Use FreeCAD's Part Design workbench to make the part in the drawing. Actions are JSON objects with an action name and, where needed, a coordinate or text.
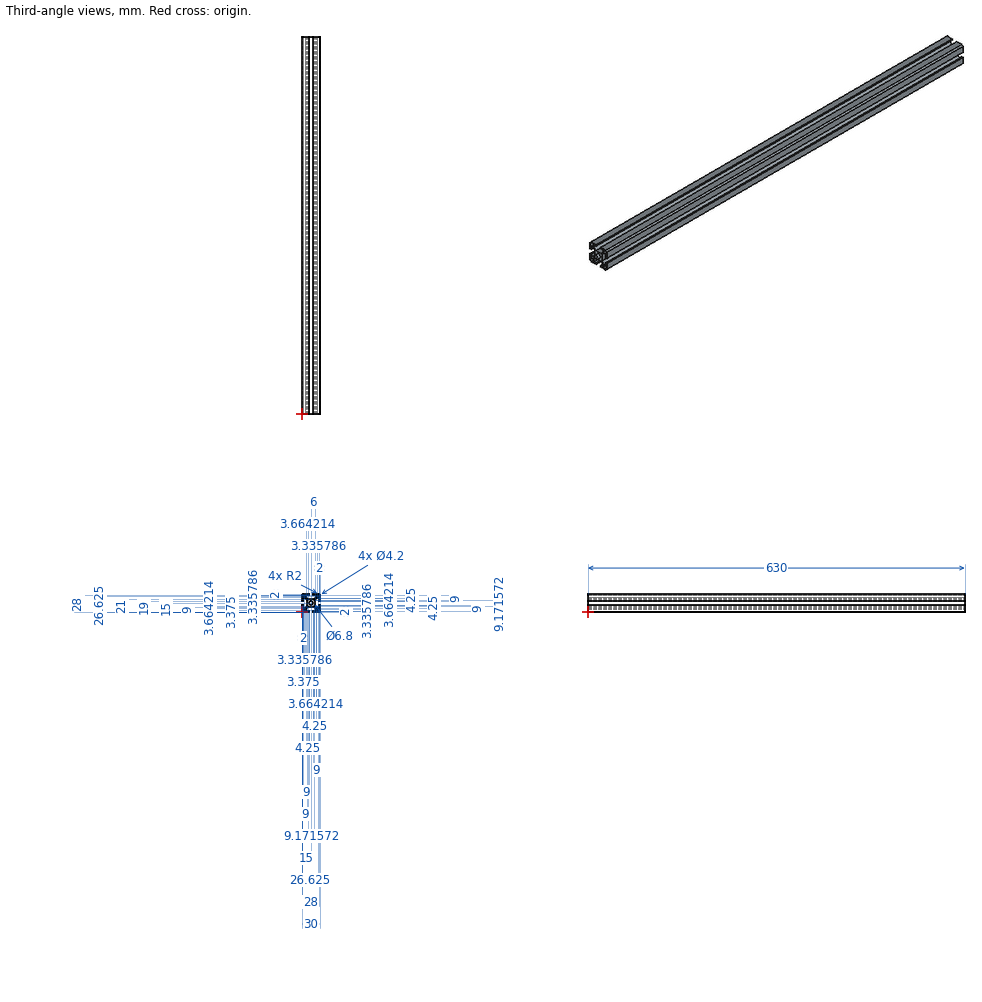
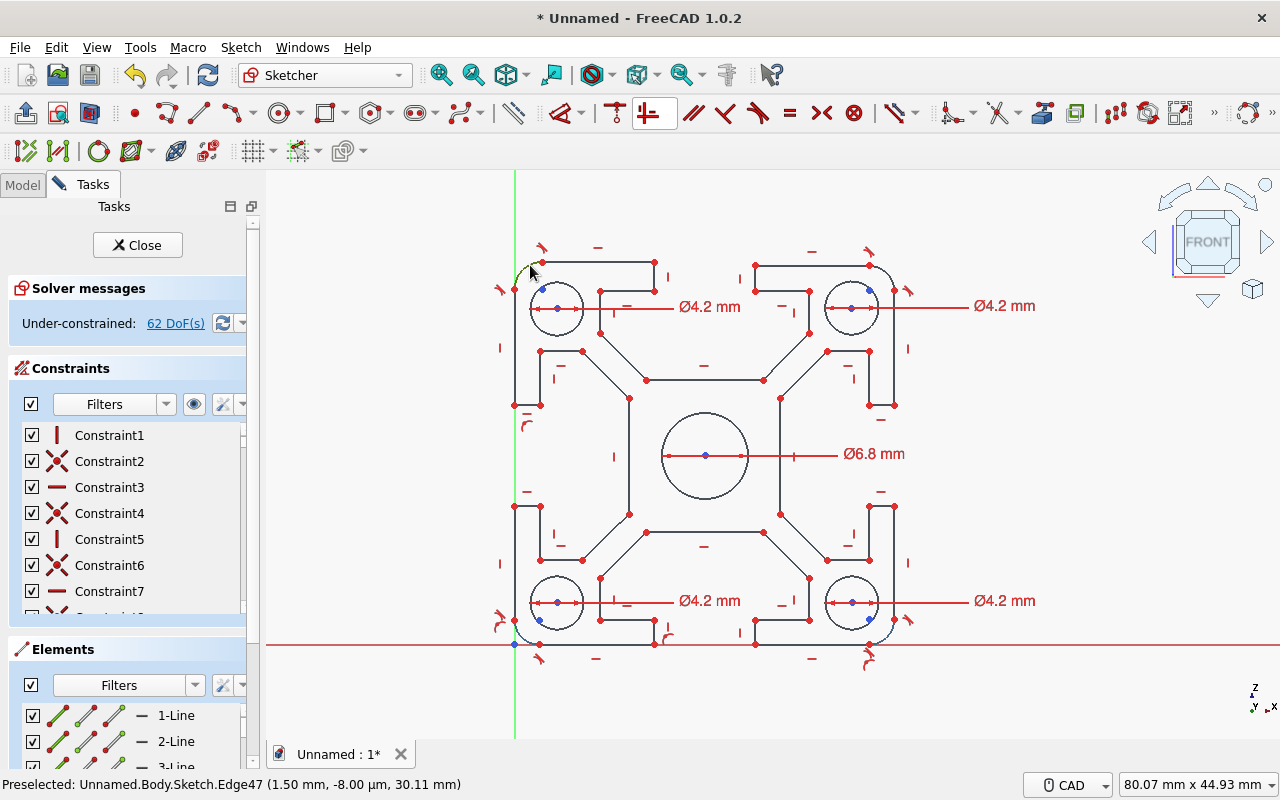
{"action": "left_click", "coordinate": [891, 280]}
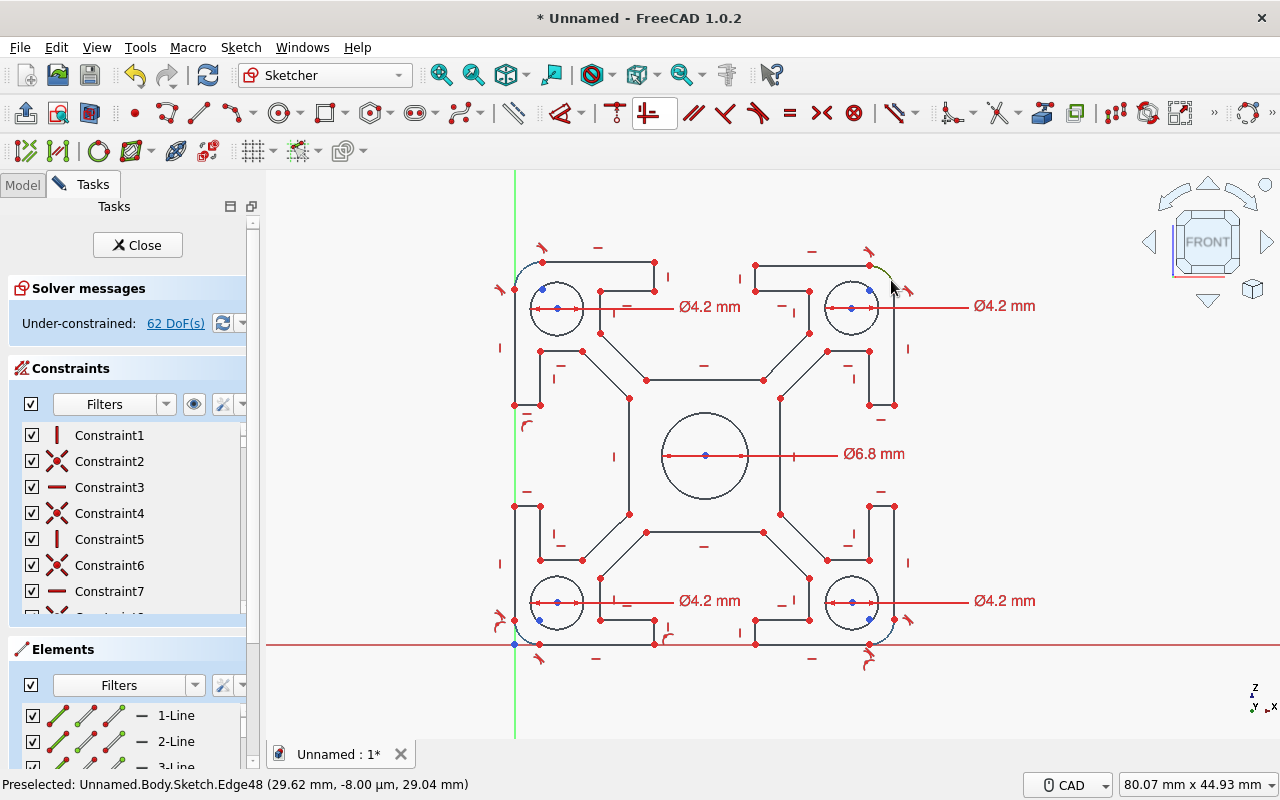
{"action": "left_click", "coordinate": [790, 114]}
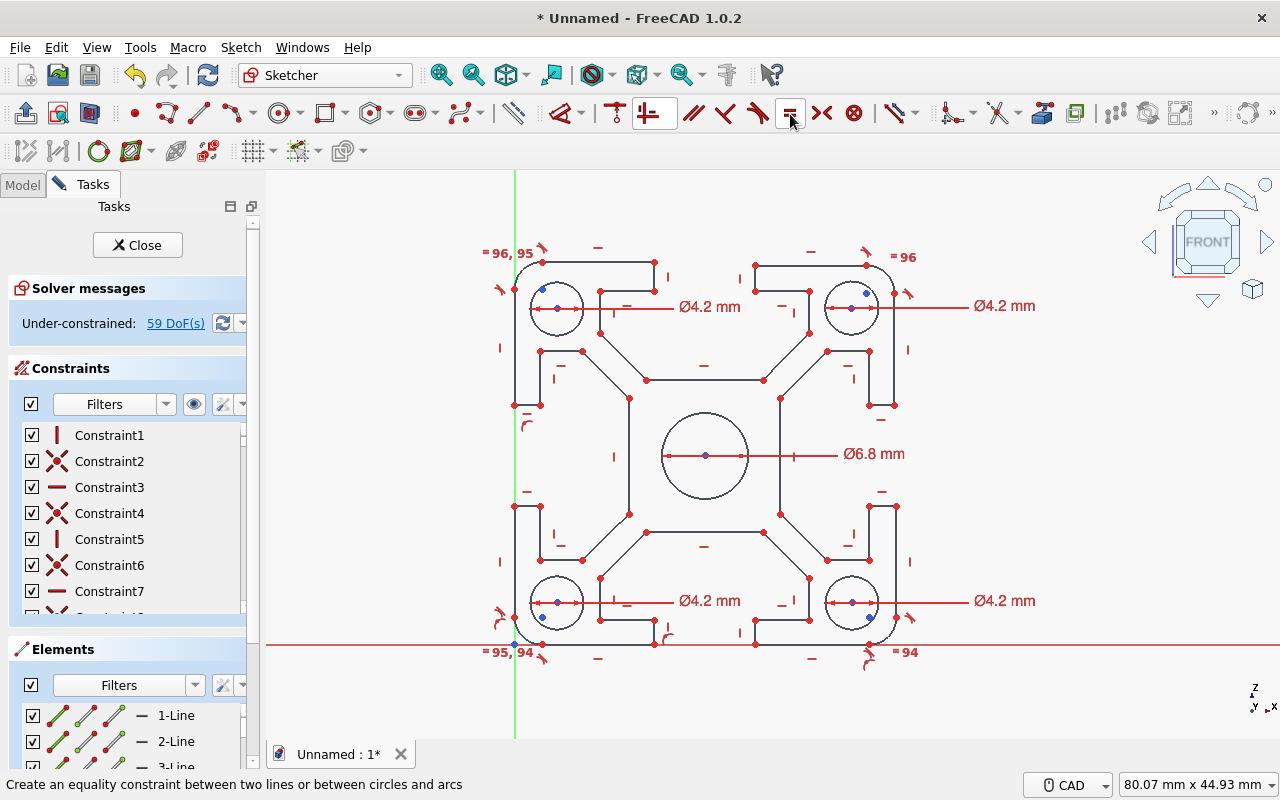
{"action": "scroll", "coordinate": [881, 642], "scroll_direction": "up", "scroll_amount": 3}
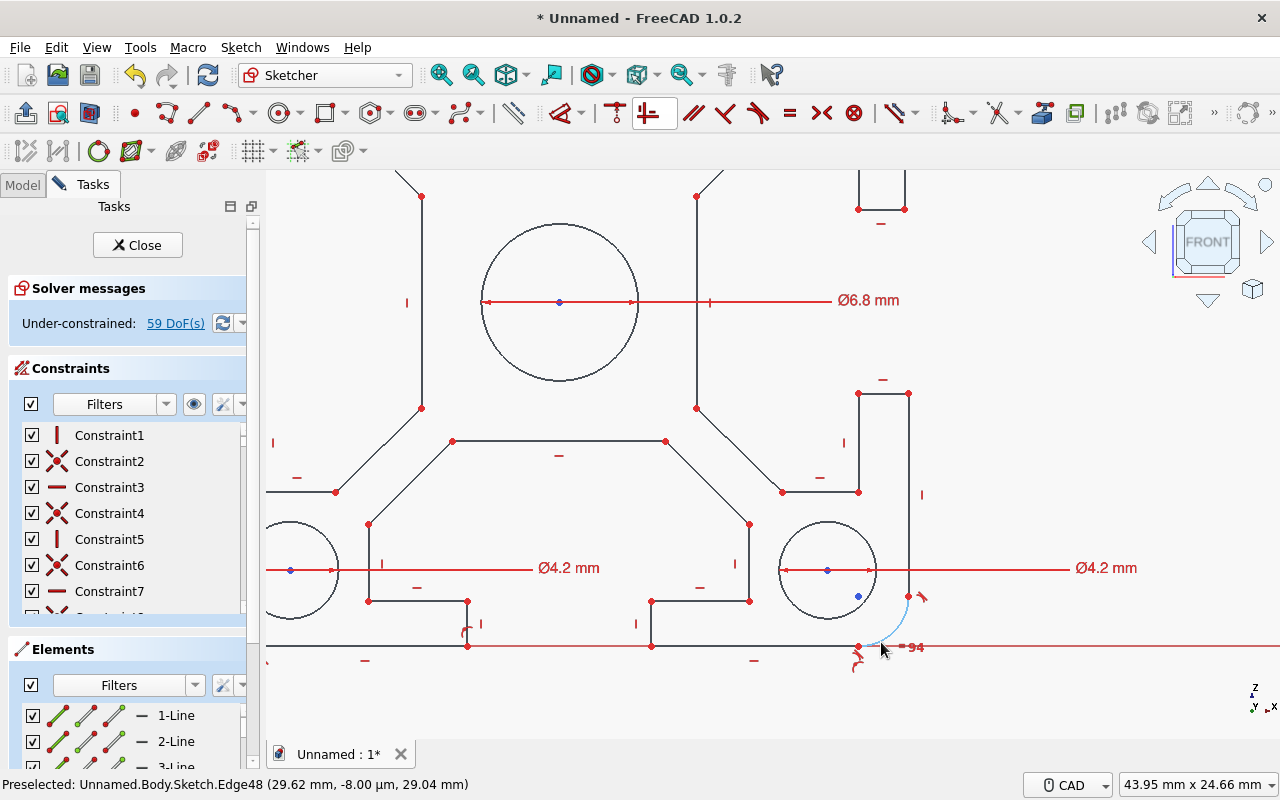
{"action": "left_click", "coordinate": [881, 641]}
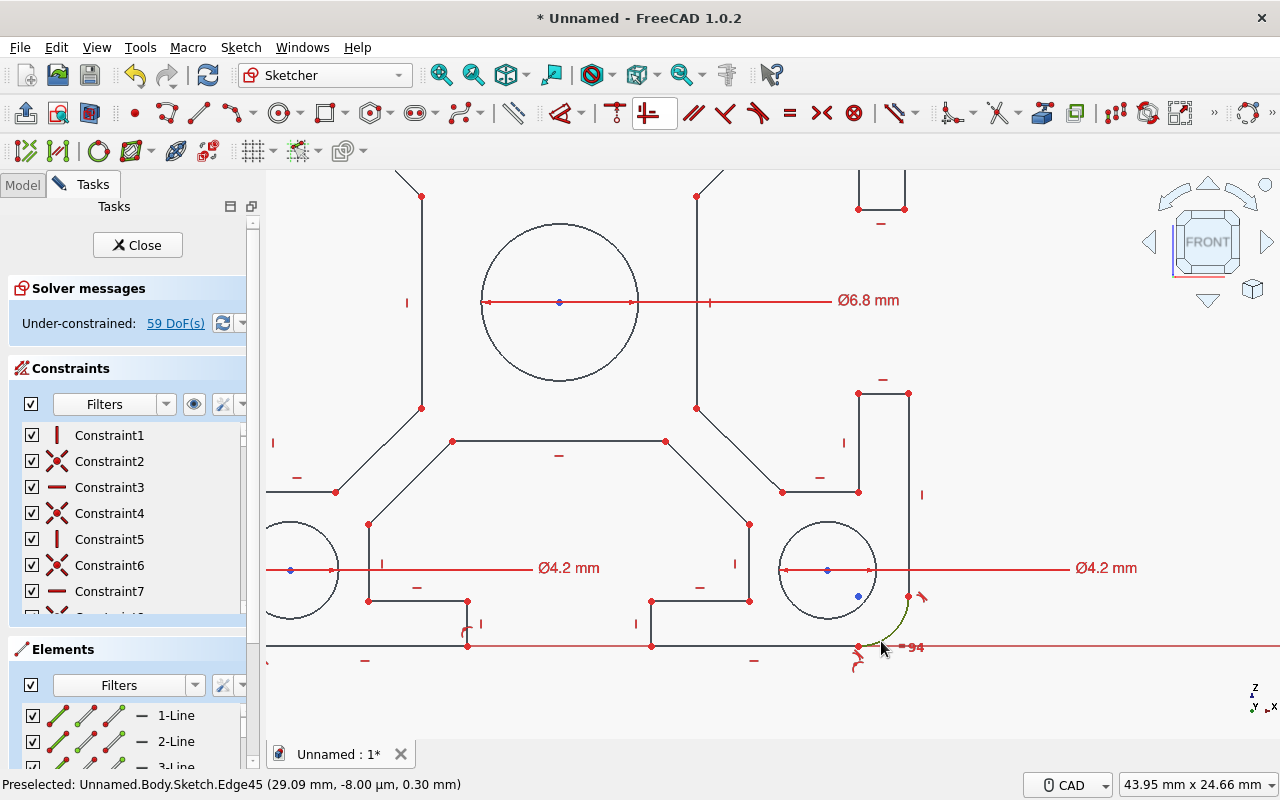
{"action": "key", "text": "k r"}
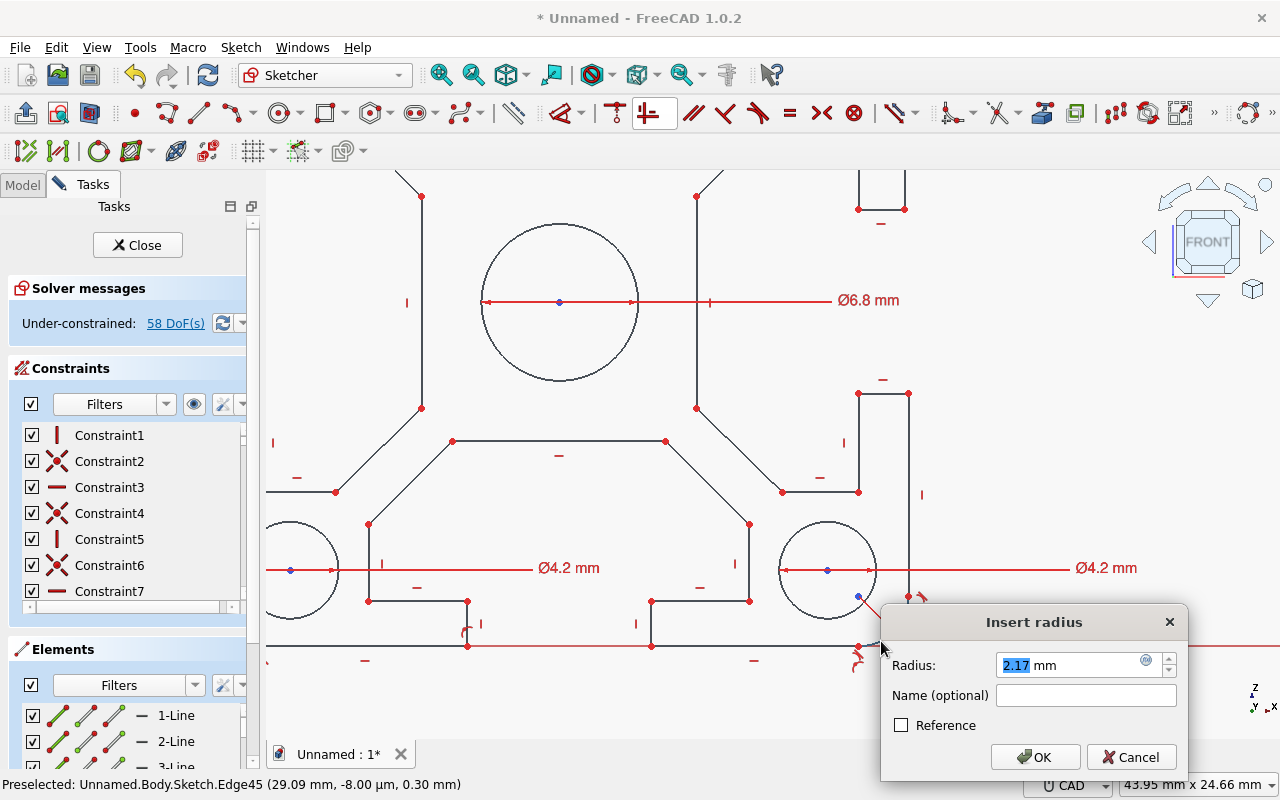
{"action": "type", "text": "2"}
{"action": "key", "text": "Return"}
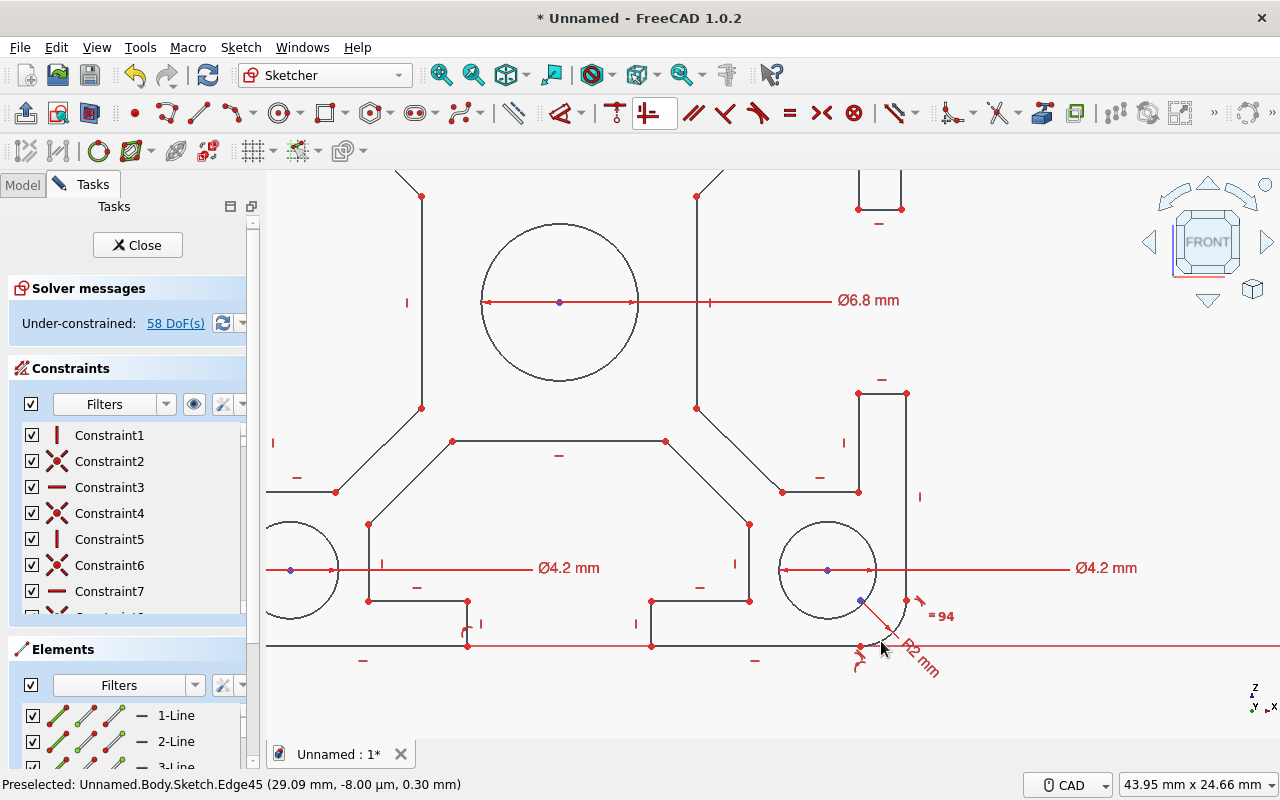
{"action": "scroll", "coordinate": [881, 642], "scroll_direction": "down", "scroll_amount": 3}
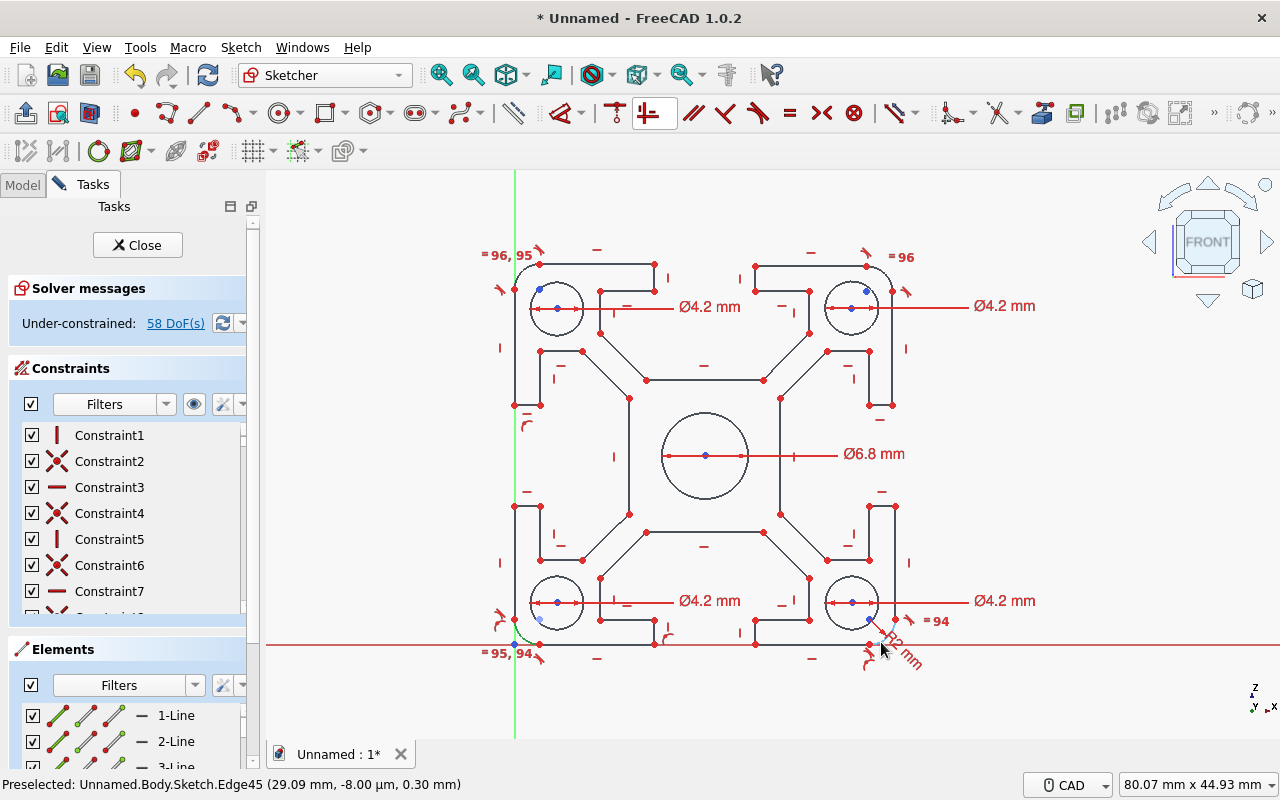
{"action": "left_click", "coordinate": [892, 326]}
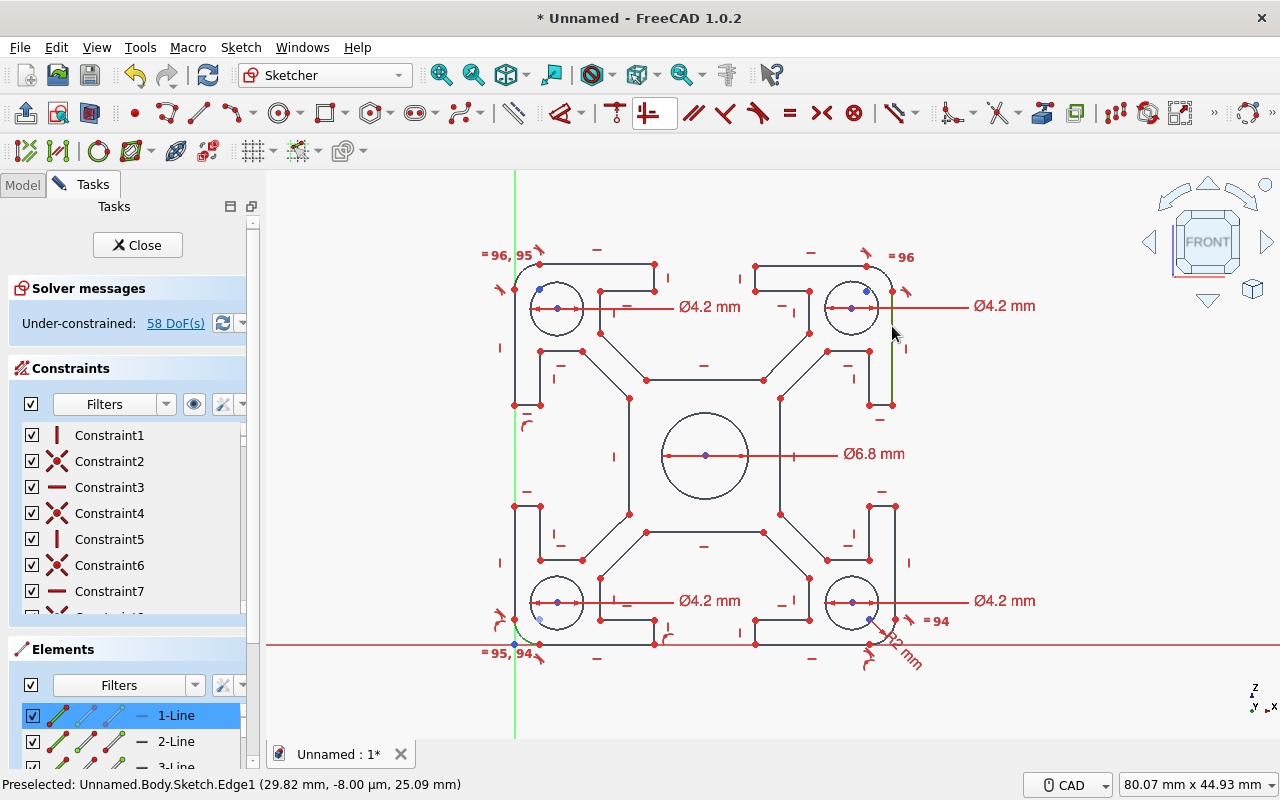
{"action": "key", "text": "i"}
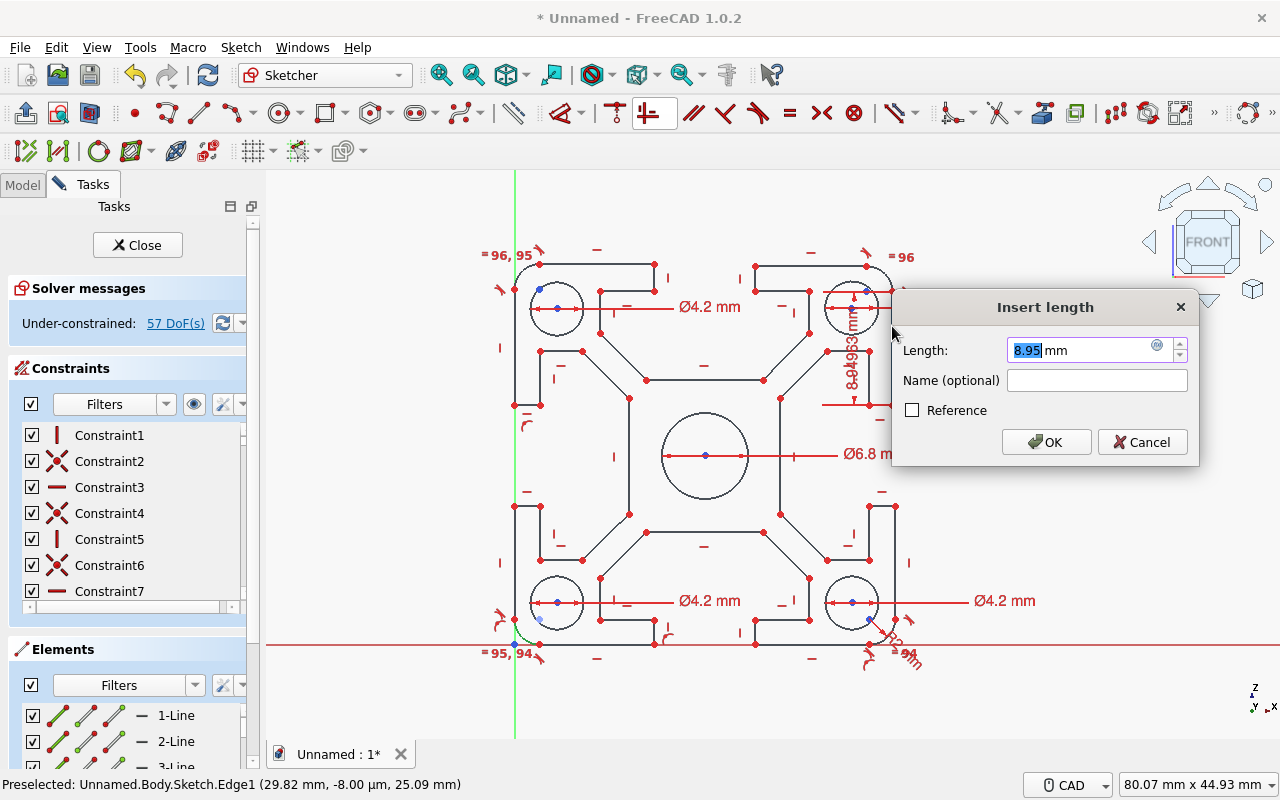
{"action": "type", "text": "9"}
{"action": "key", "text": "Return"}